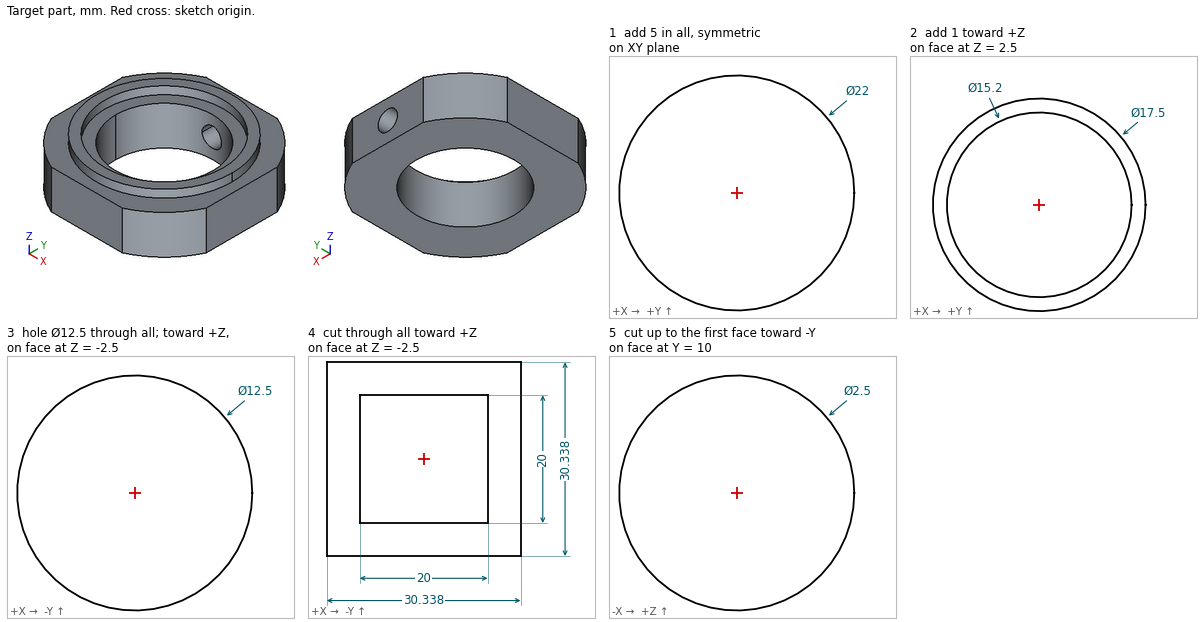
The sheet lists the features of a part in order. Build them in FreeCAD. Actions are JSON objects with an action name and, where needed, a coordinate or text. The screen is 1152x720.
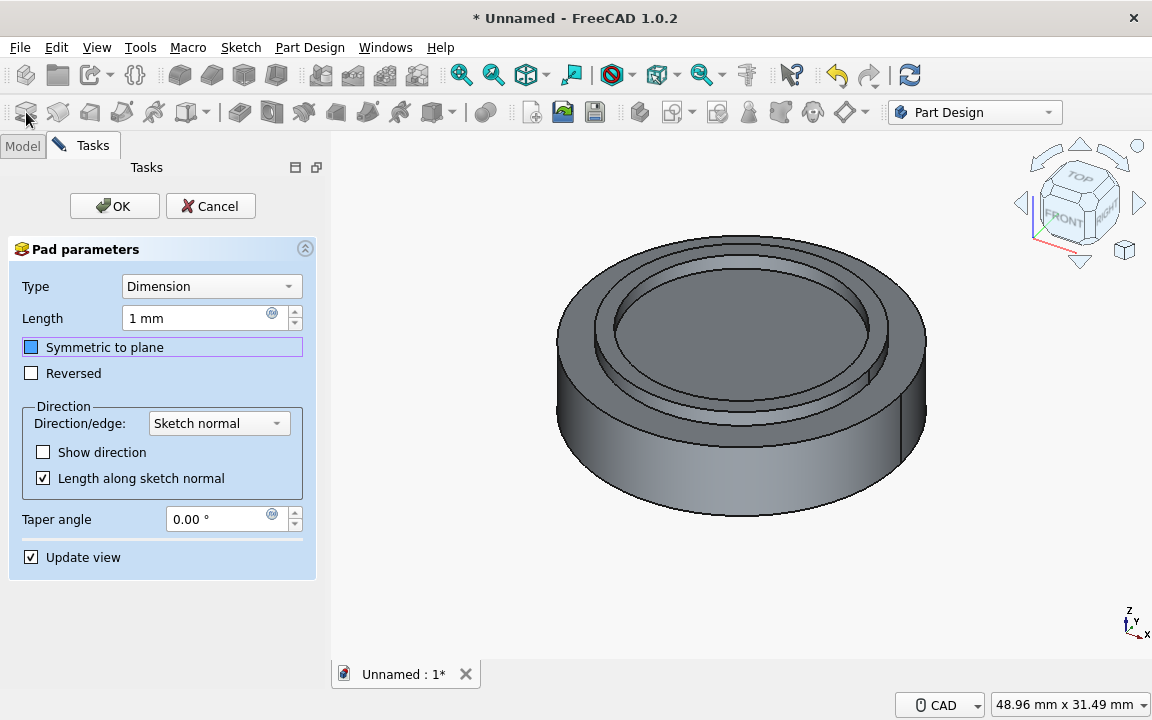
{"action": "left_click", "coordinate": [115, 206]}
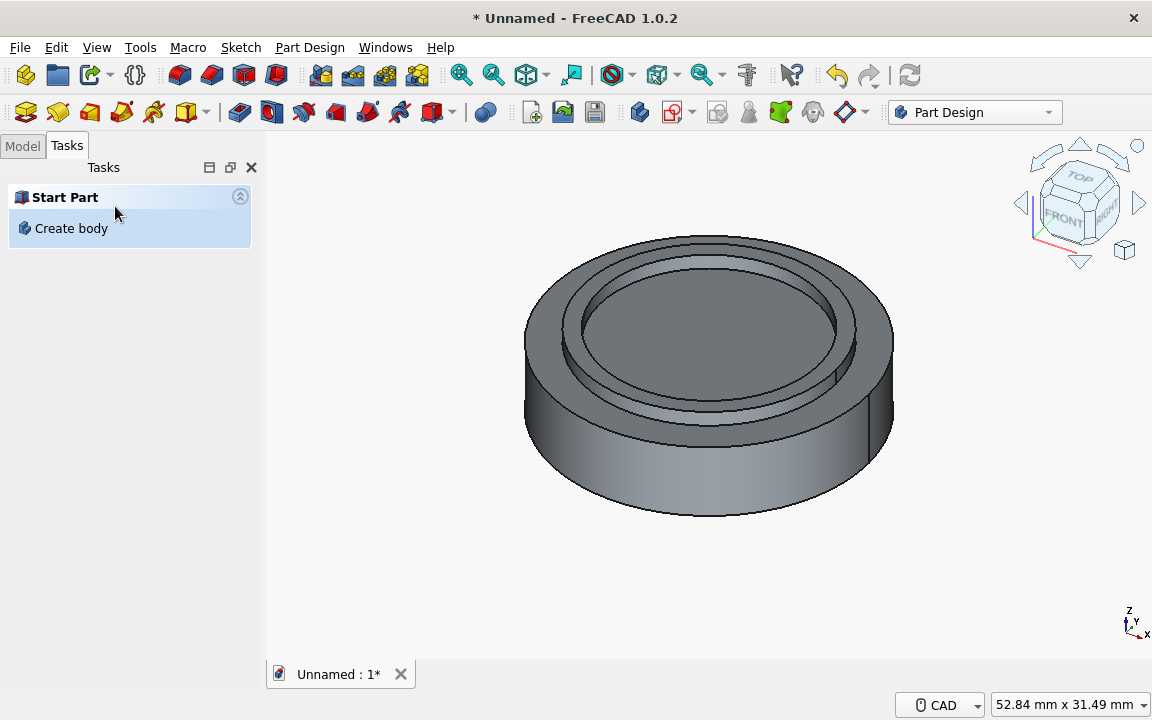
{"action": "key", "text": "5"}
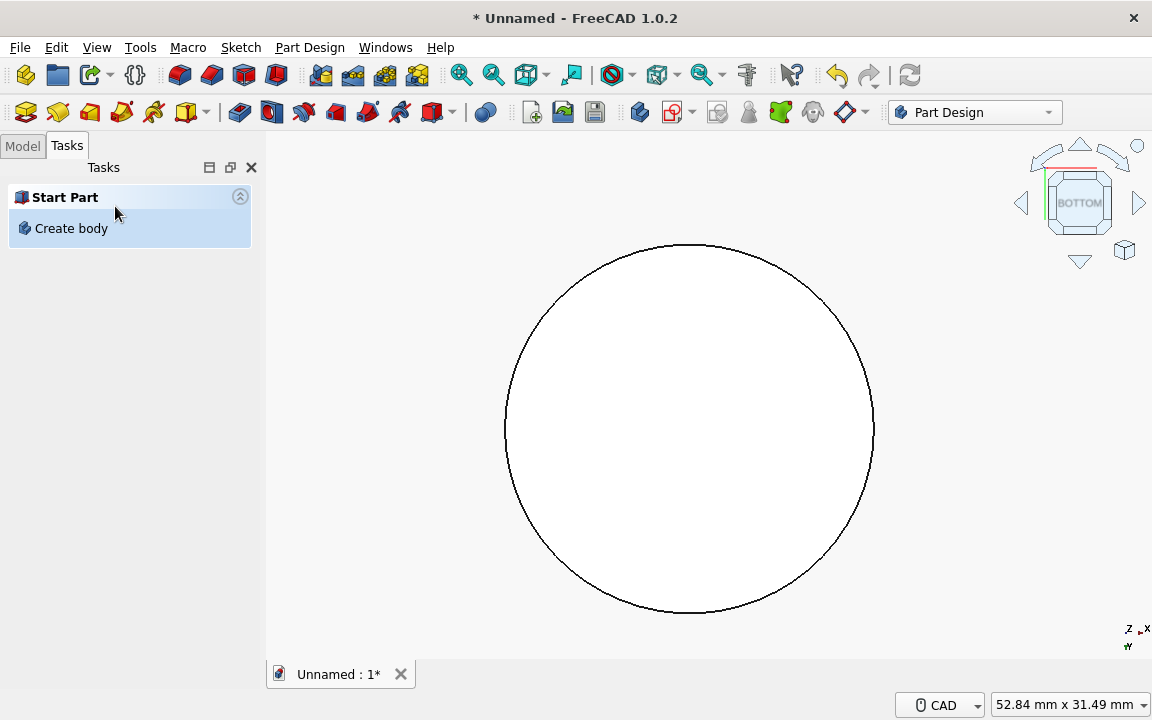
{"action": "left_click", "coordinate": [689, 428]}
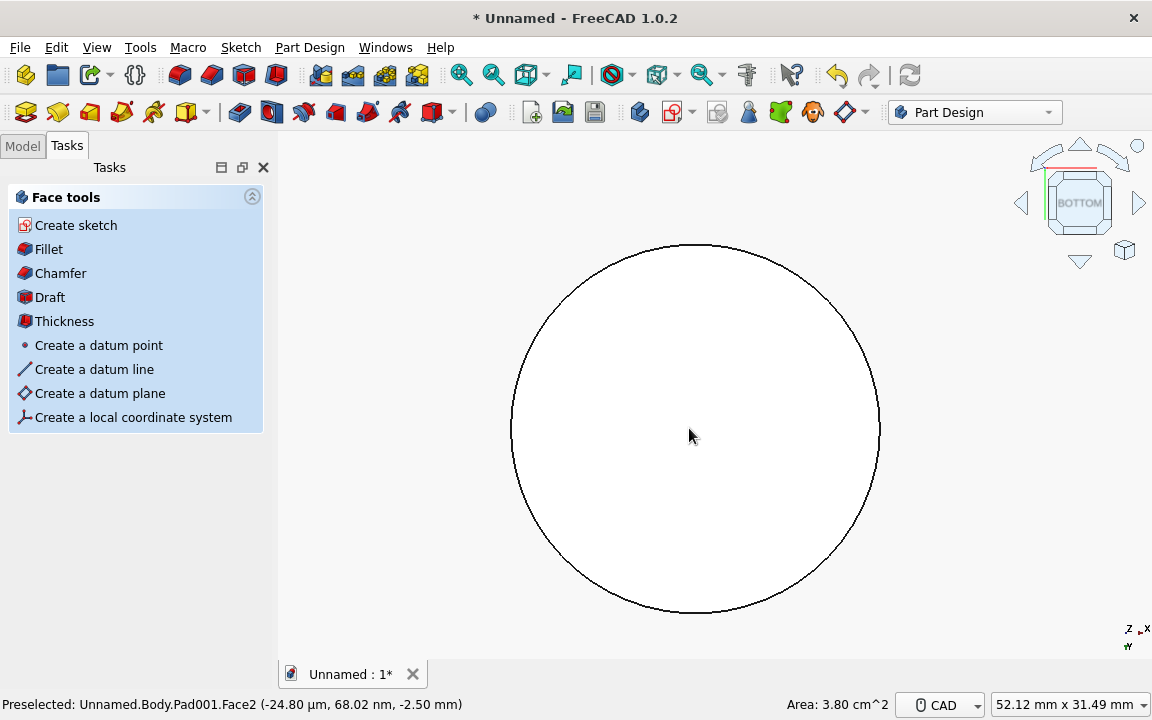
{"action": "left_click", "coordinate": [672, 112]}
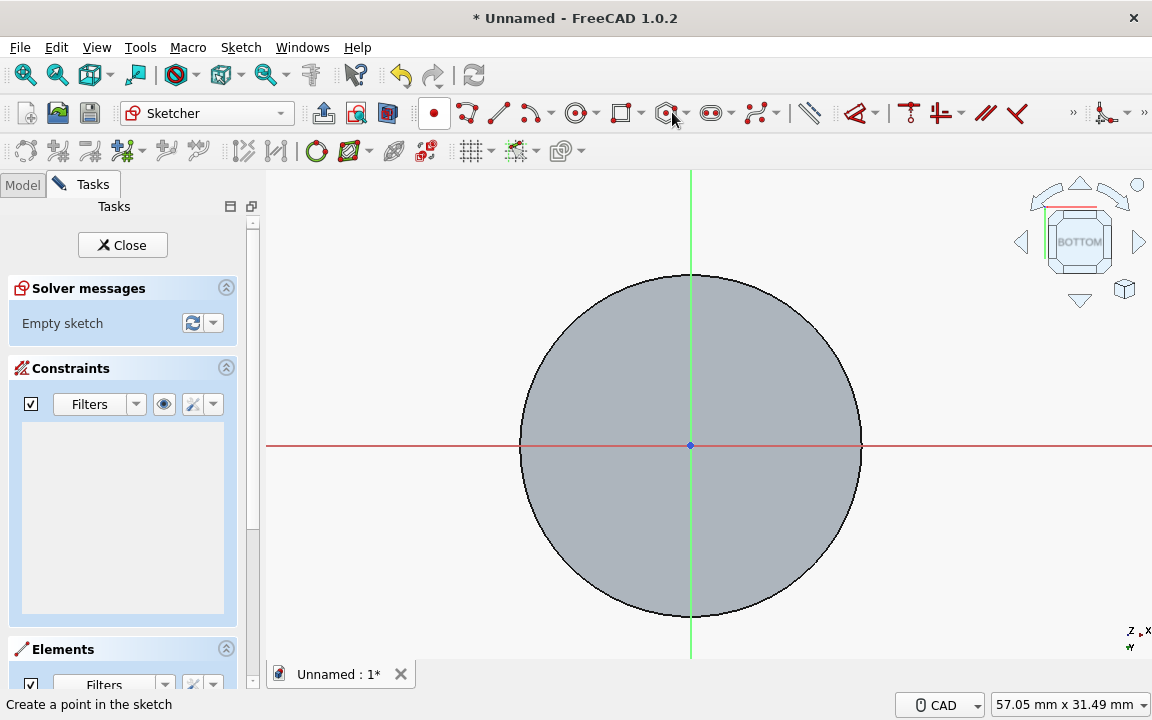
{"action": "scroll", "coordinate": [793, 510], "scroll_direction": "up", "scroll_amount": 2}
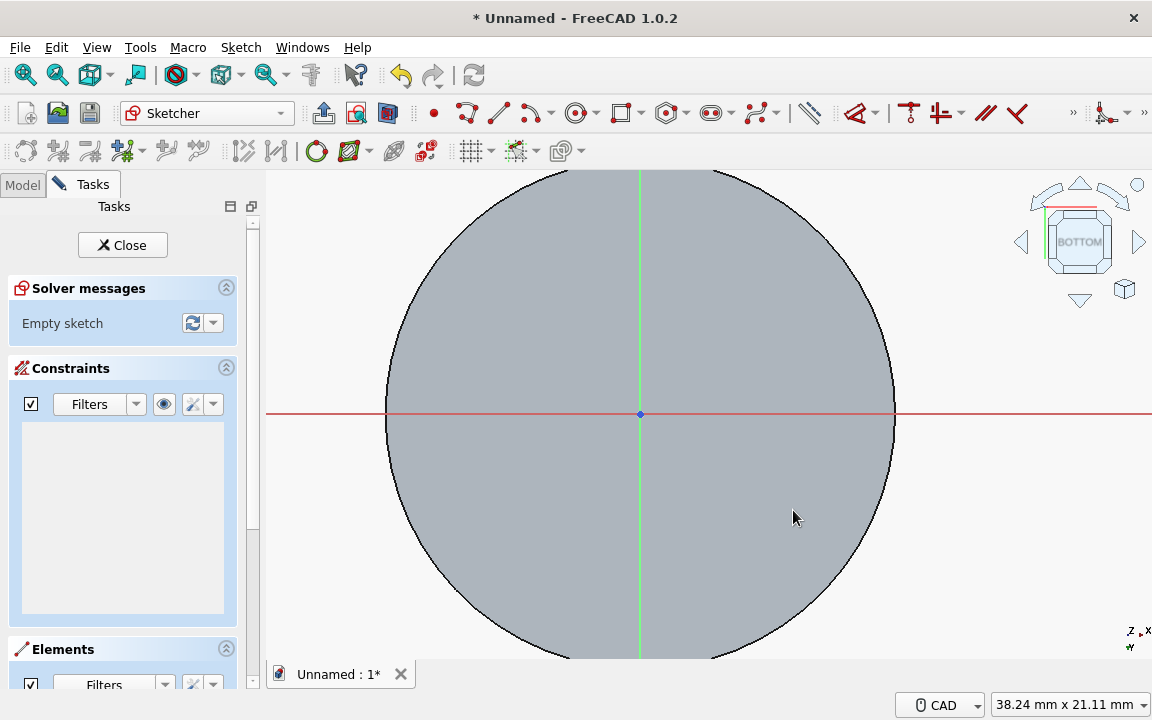
{"action": "left_click", "coordinate": [576, 114]}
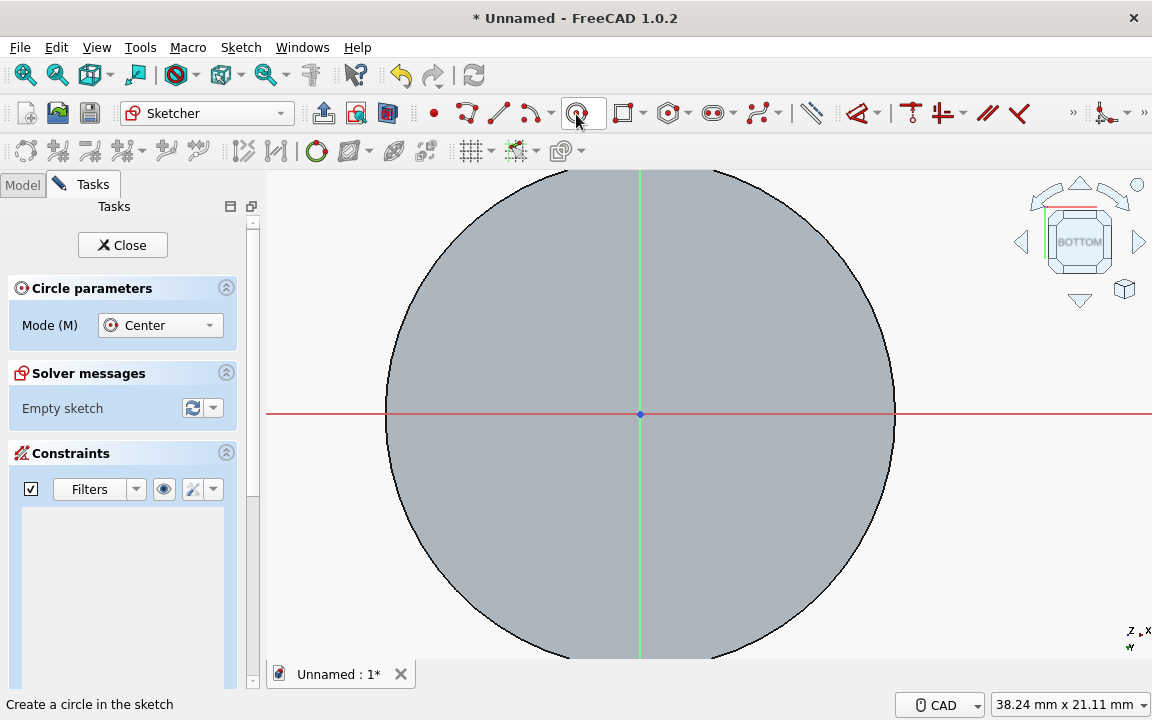
{"action": "left_click", "coordinate": [640, 414]}
{"action": "mouse_move", "coordinate": [743, 312]}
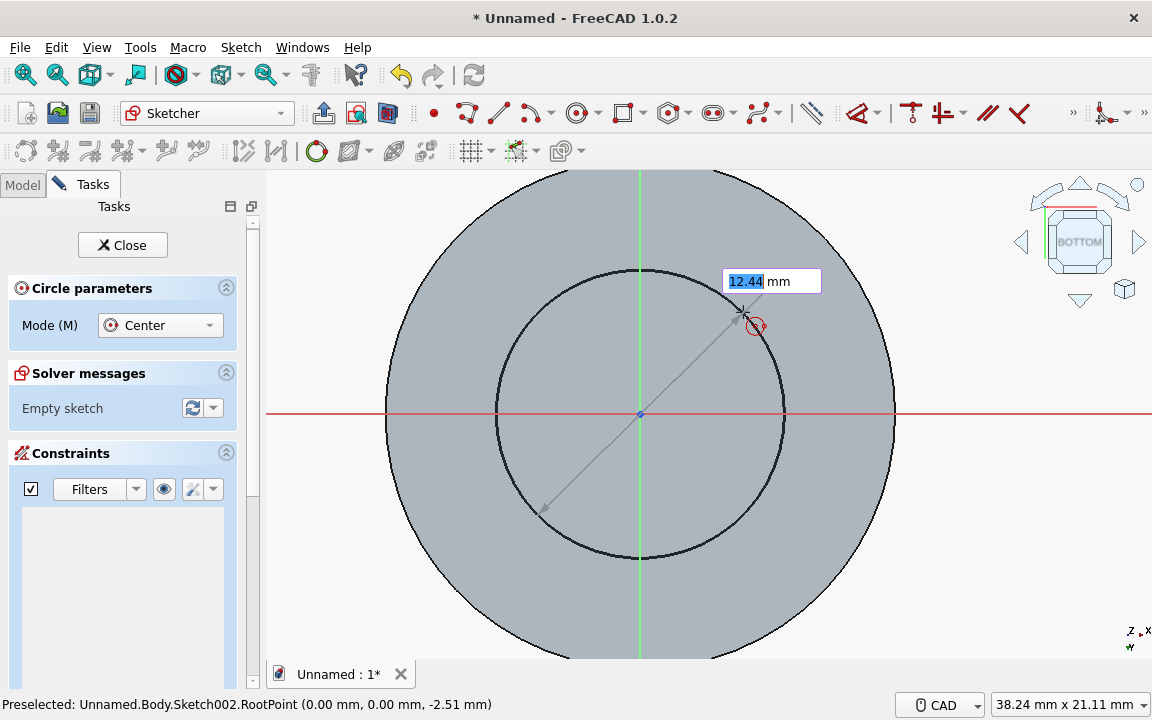
{"action": "type", "text": "12.5"}
{"action": "key", "text": "Return"}
{"action": "key", "text": "Escape"}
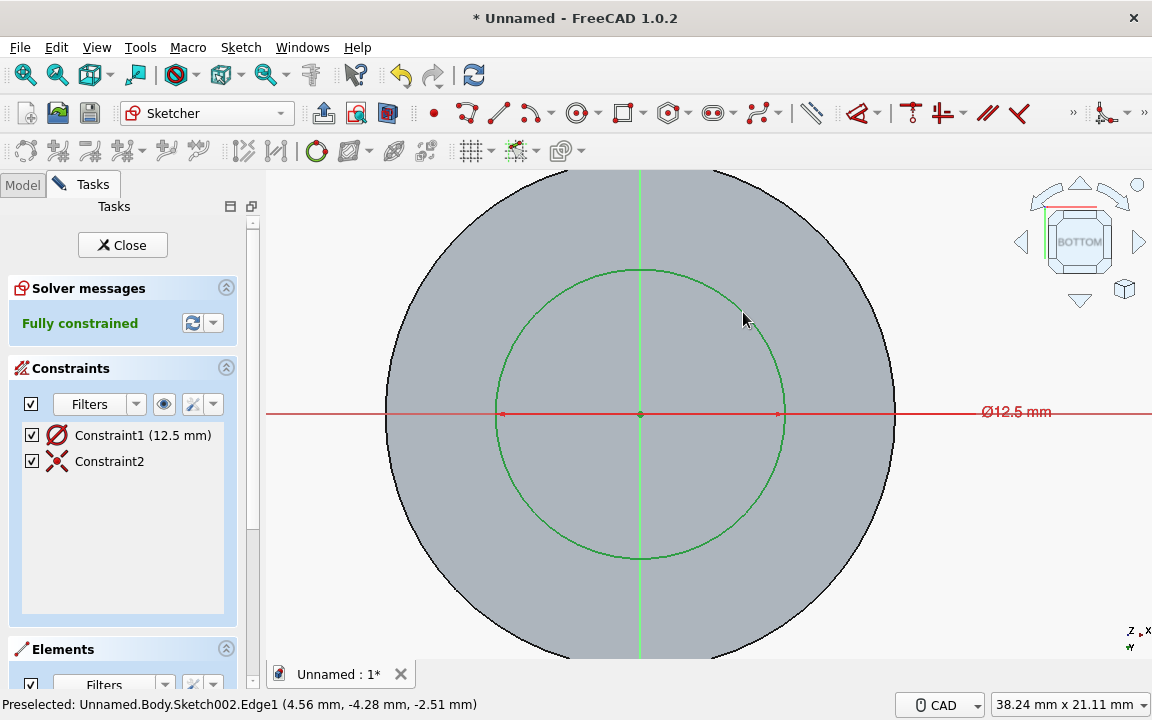
{"action": "left_click", "coordinate": [123, 245]}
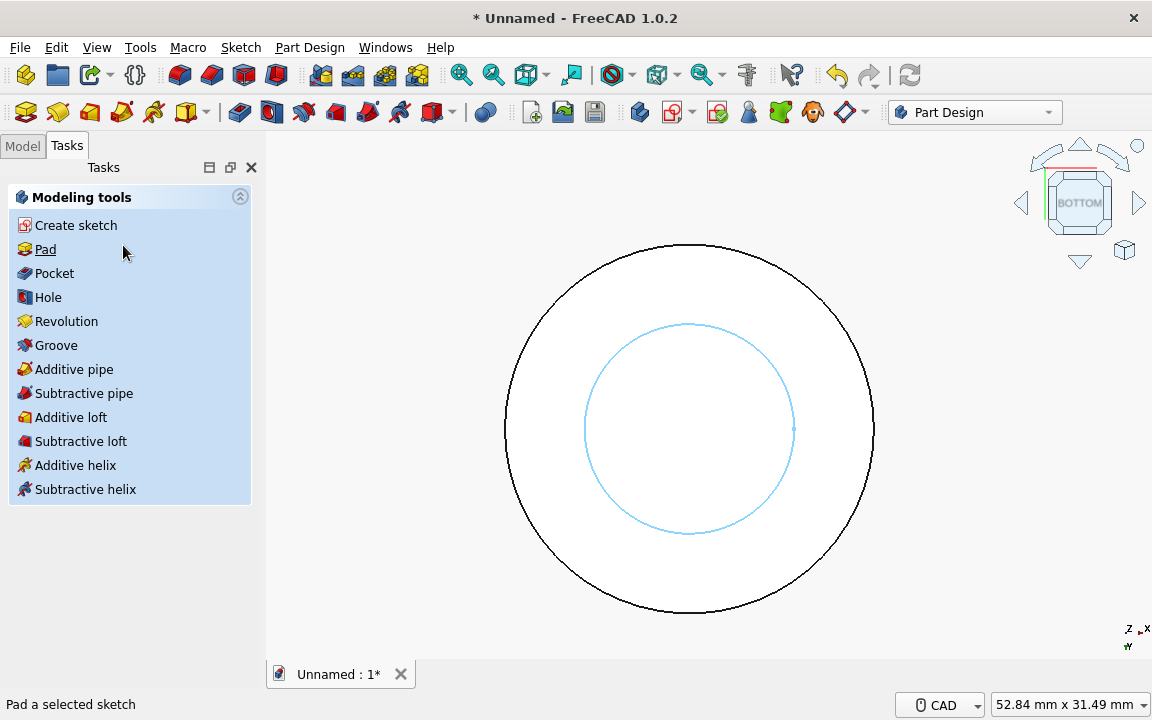
{"action": "left_click", "coordinate": [272, 112]}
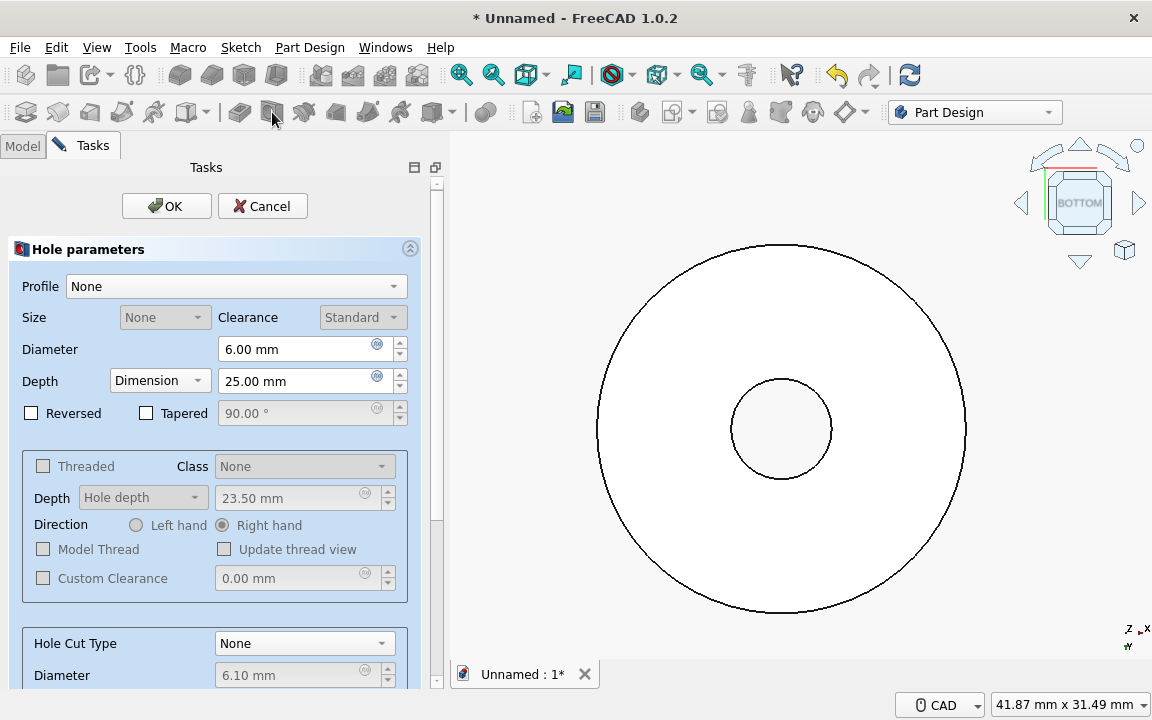
{"action": "triple_click", "coordinate": [305, 349]}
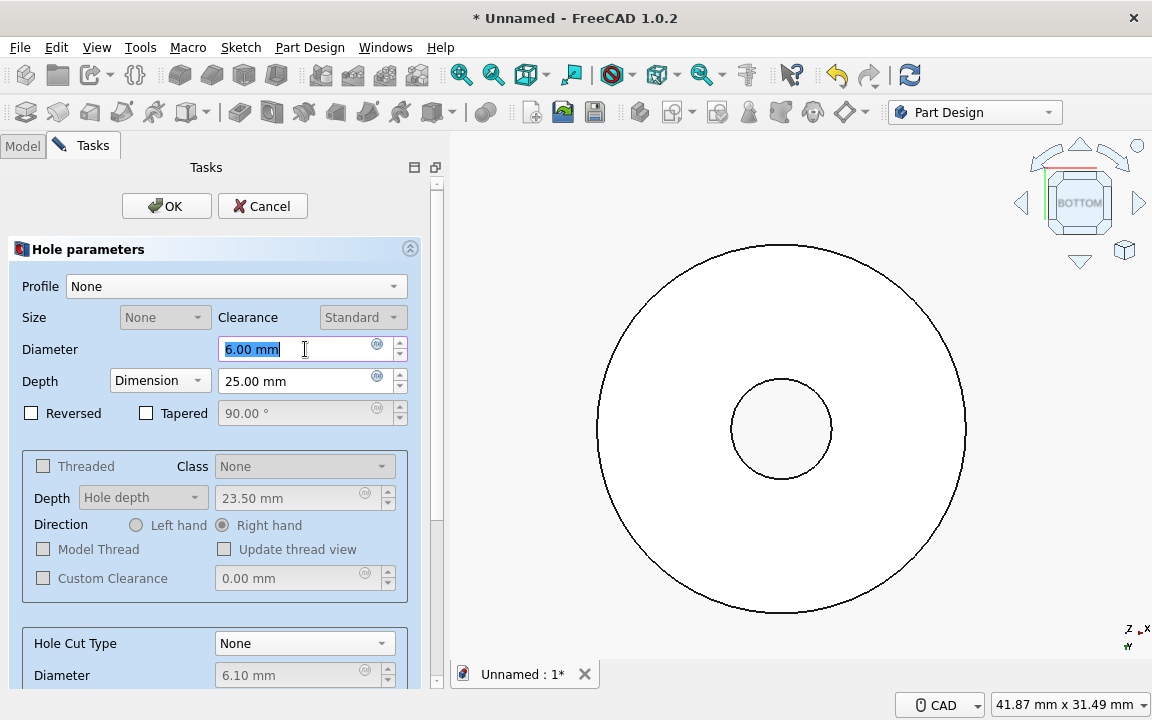
{"action": "type", "text": "12.5"}
{"action": "key", "text": "Tab"}